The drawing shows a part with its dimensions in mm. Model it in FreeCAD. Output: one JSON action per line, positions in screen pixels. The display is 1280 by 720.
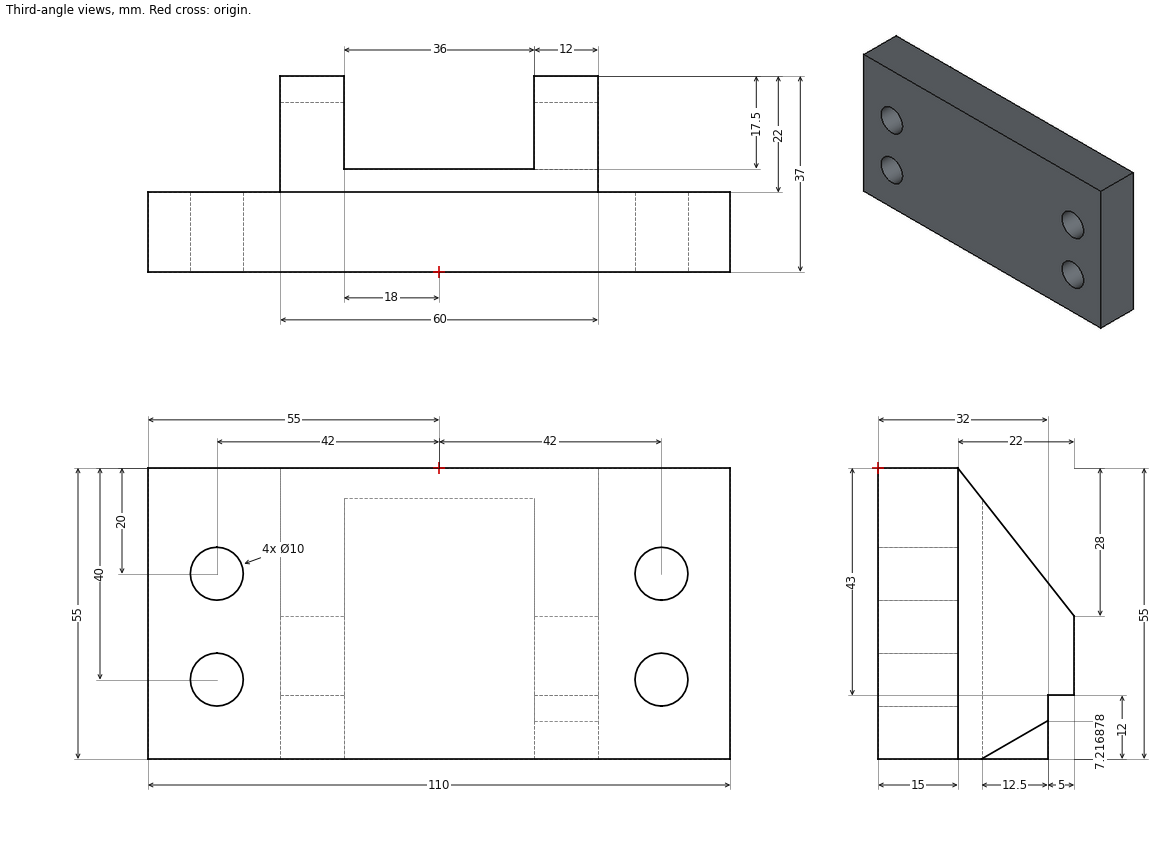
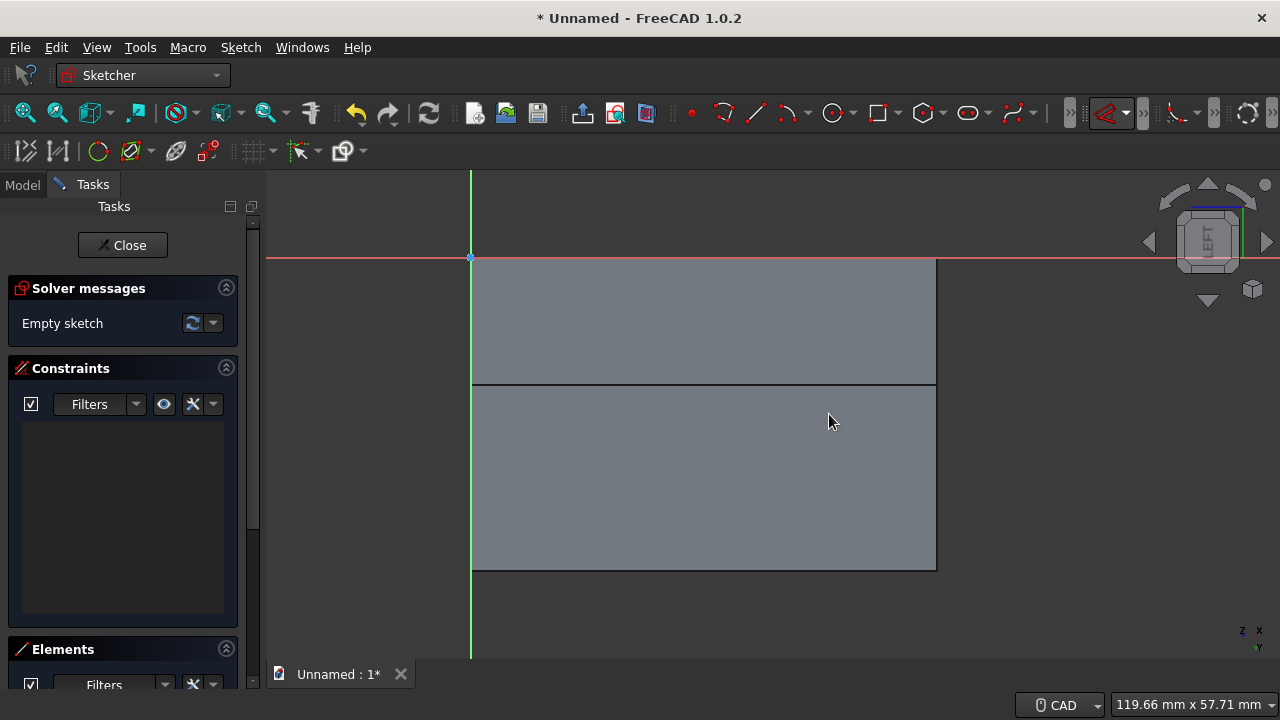
{"action": "left_click", "coordinate": [724, 114]}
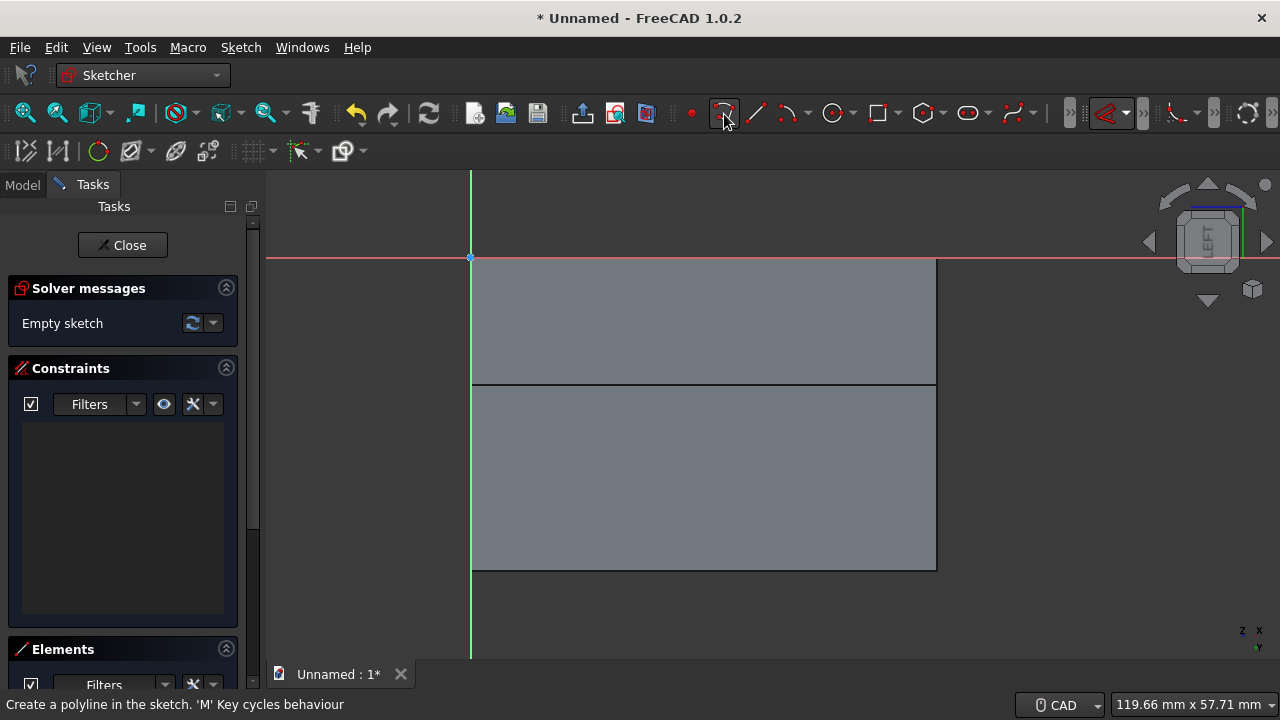
{"action": "left_click", "coordinate": [471, 385]}
{"action": "left_click", "coordinate": [480, 571]}
{"action": "left_click", "coordinate": [708, 571]}
{"action": "left_click", "coordinate": [471, 386]}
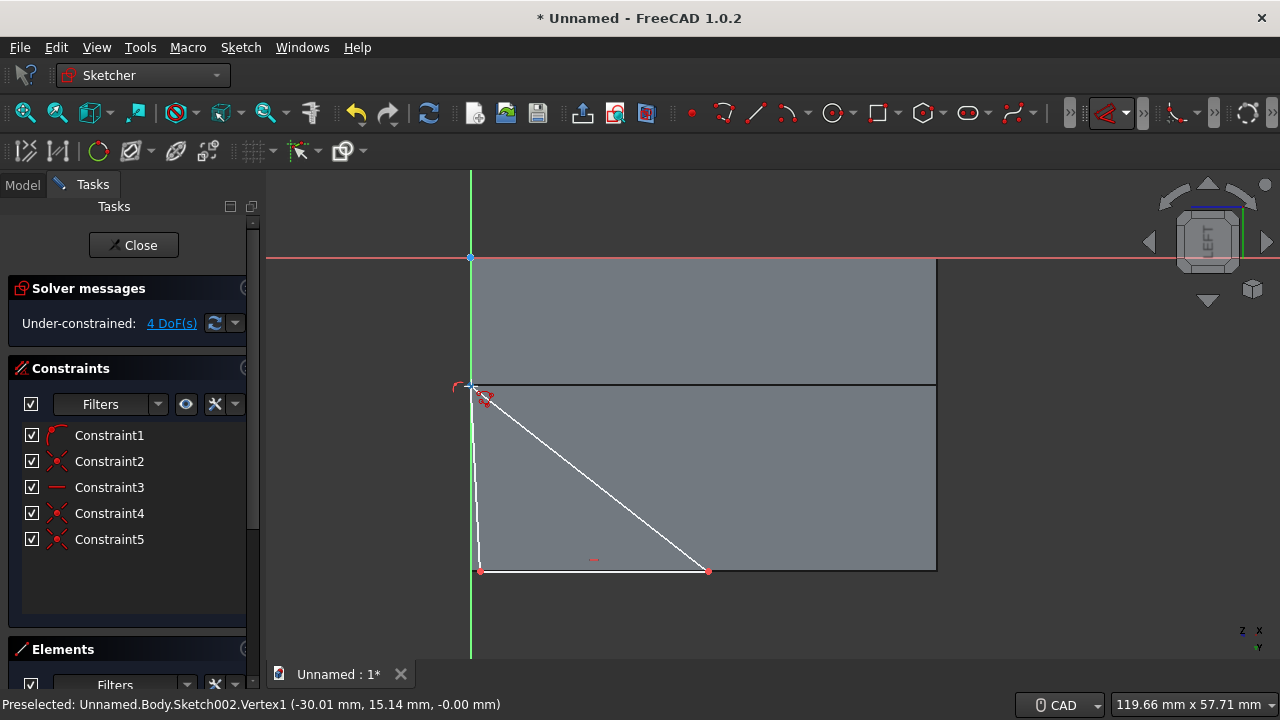
{"action": "left_click", "coordinate": [878, 114]}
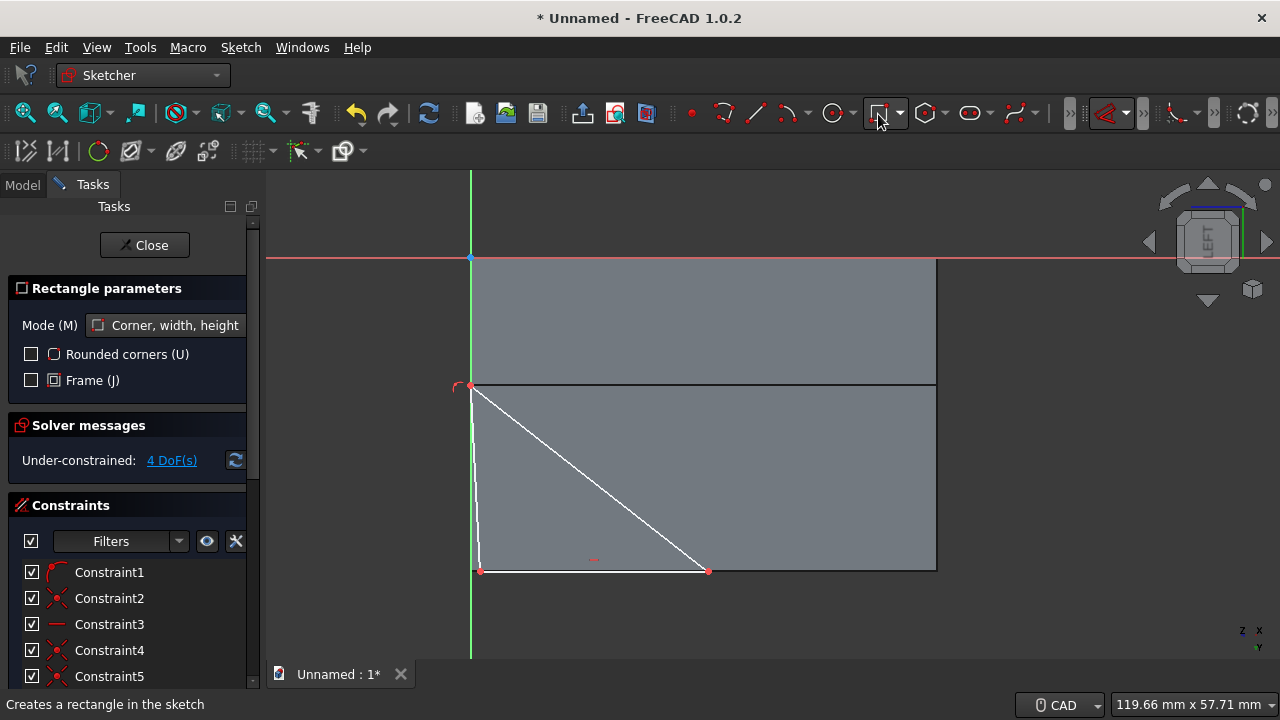
{"action": "left_click", "coordinate": [835, 529]}
{"action": "left_click", "coordinate": [937, 571]}
{"action": "key", "text": "Escape"}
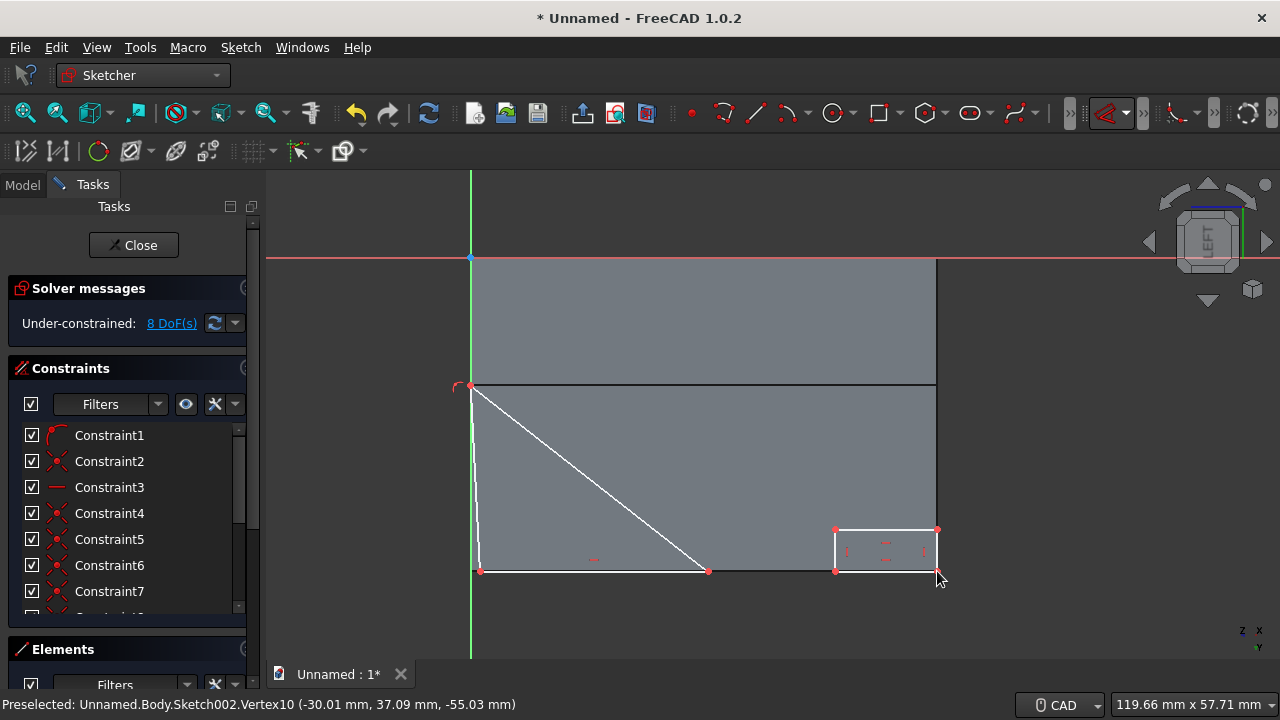
{"action": "left_click", "coordinate": [473, 442]}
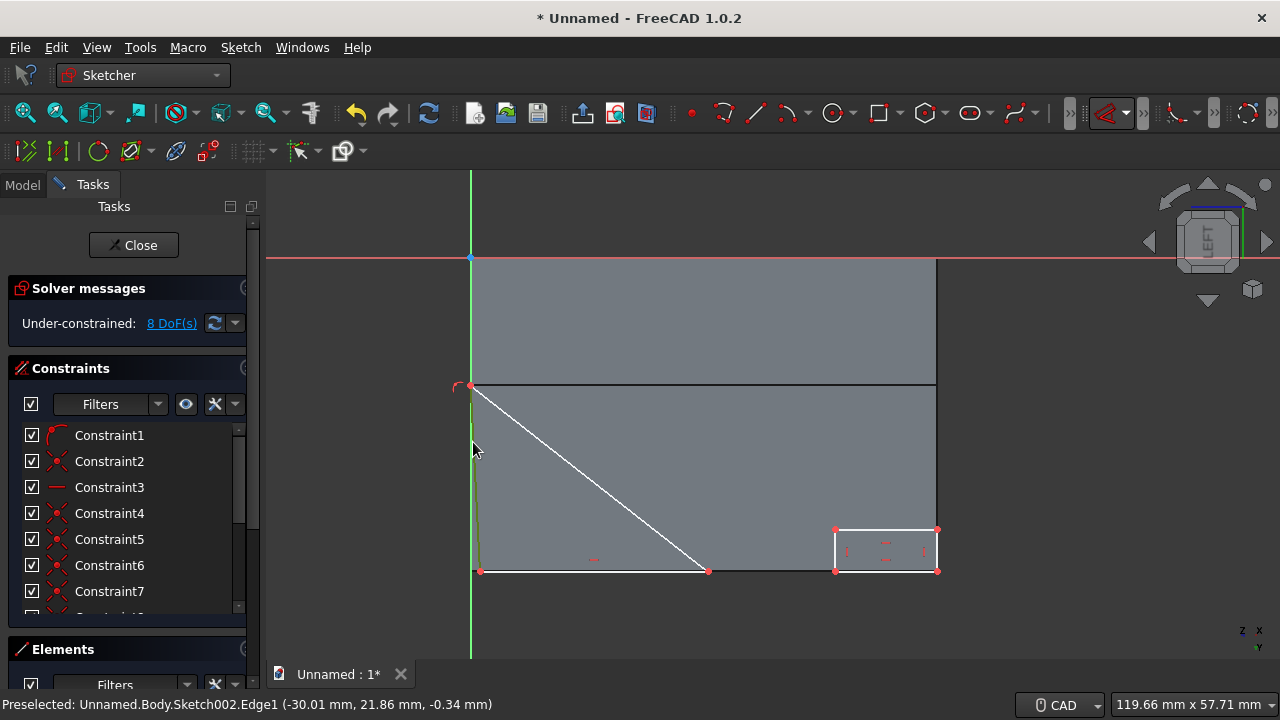
{"action": "key", "text": "v"}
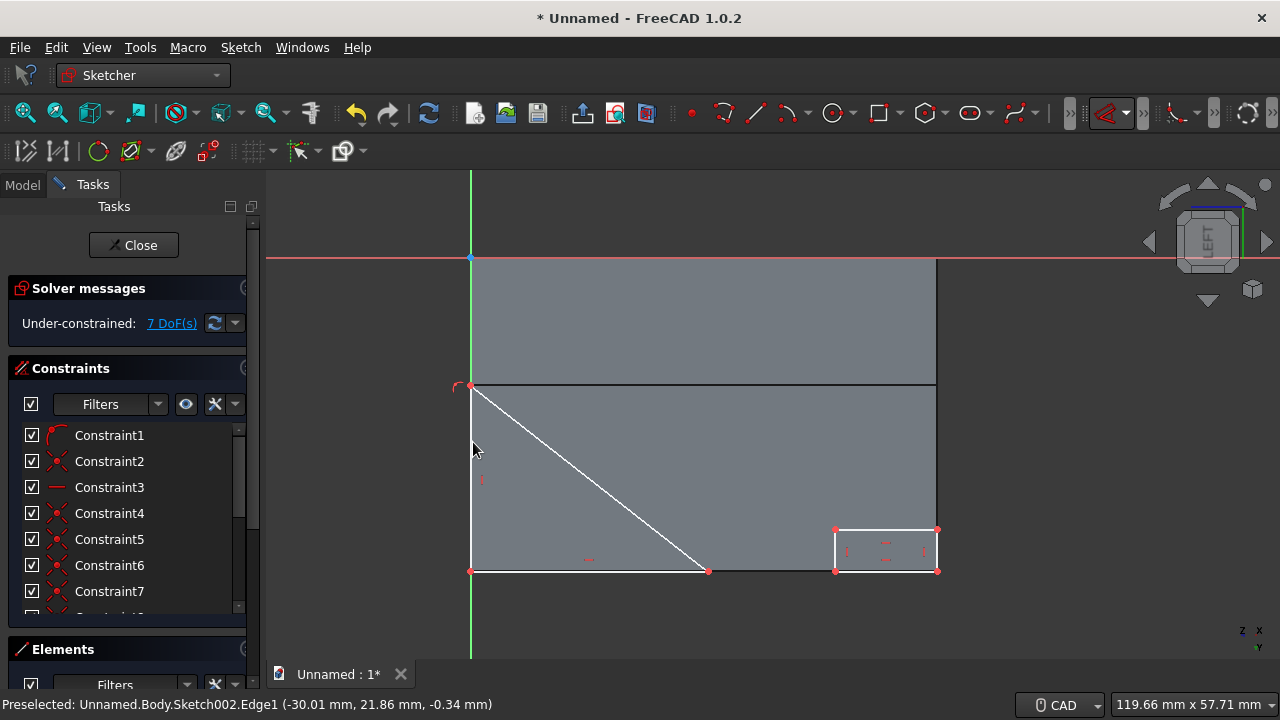
{"action": "left_click", "coordinate": [835, 543]}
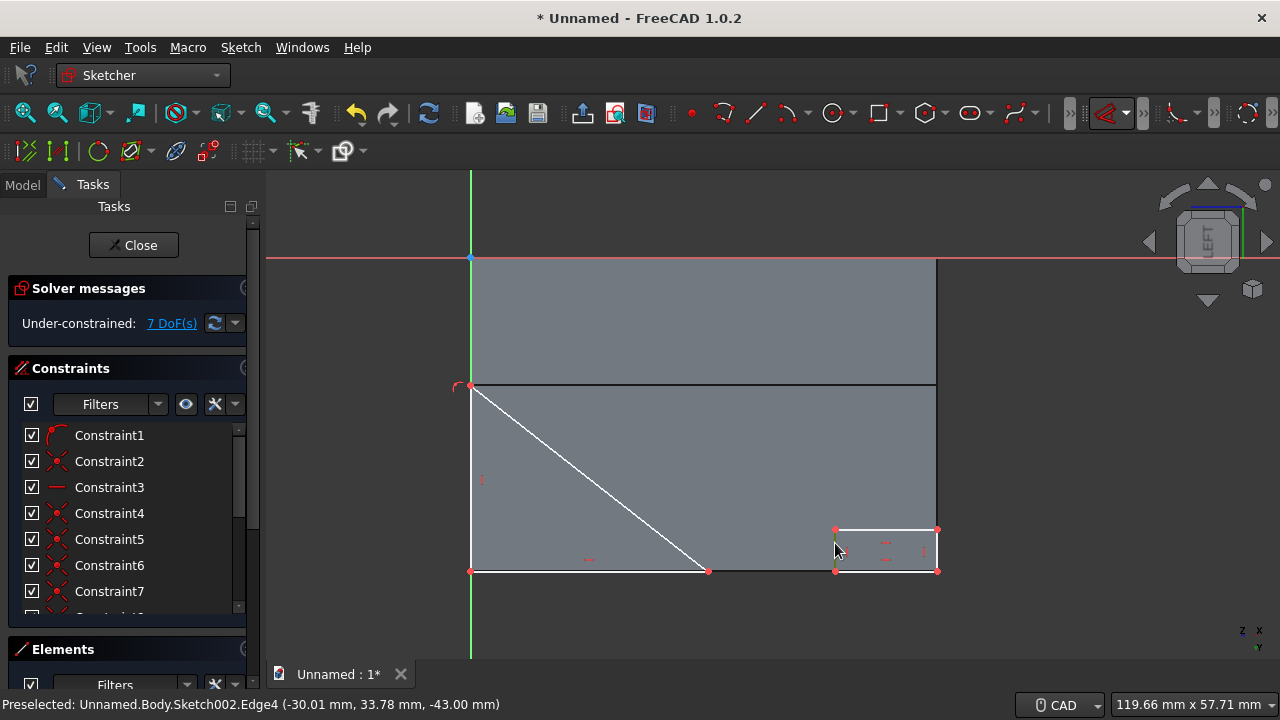
{"action": "left_click", "coordinate": [1128, 114]}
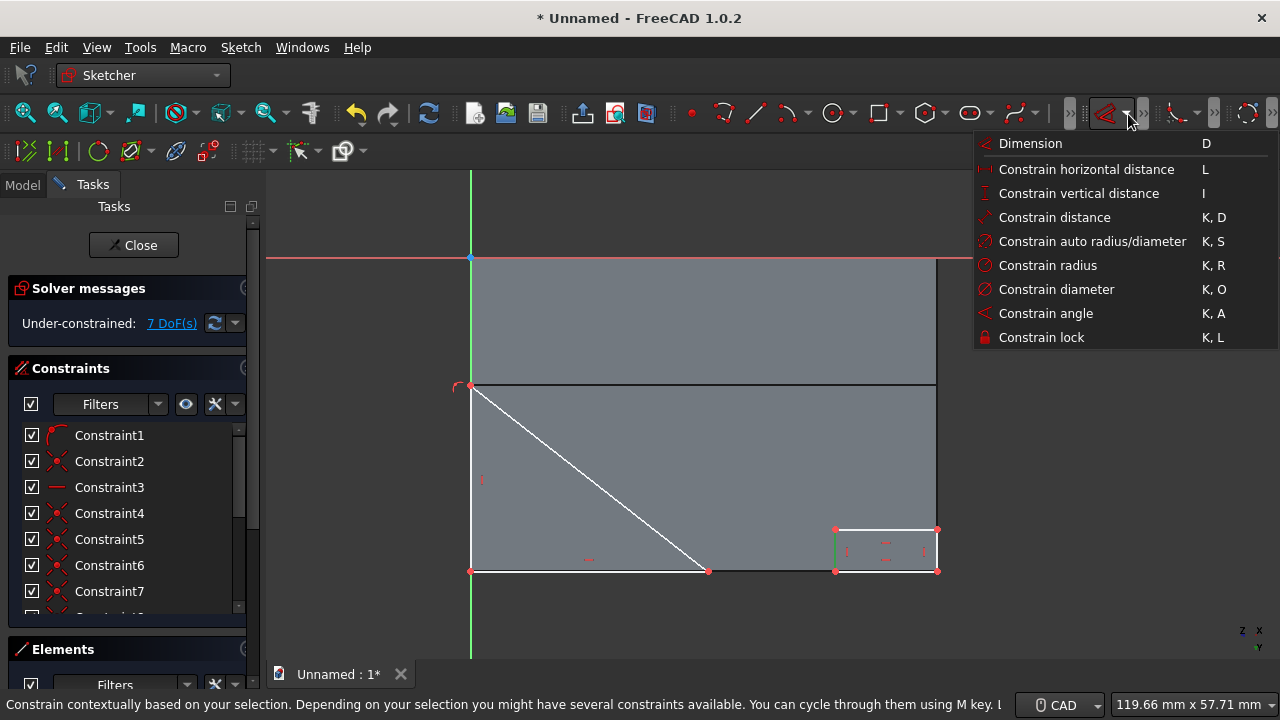
{"action": "left_click", "coordinate": [1126, 193]}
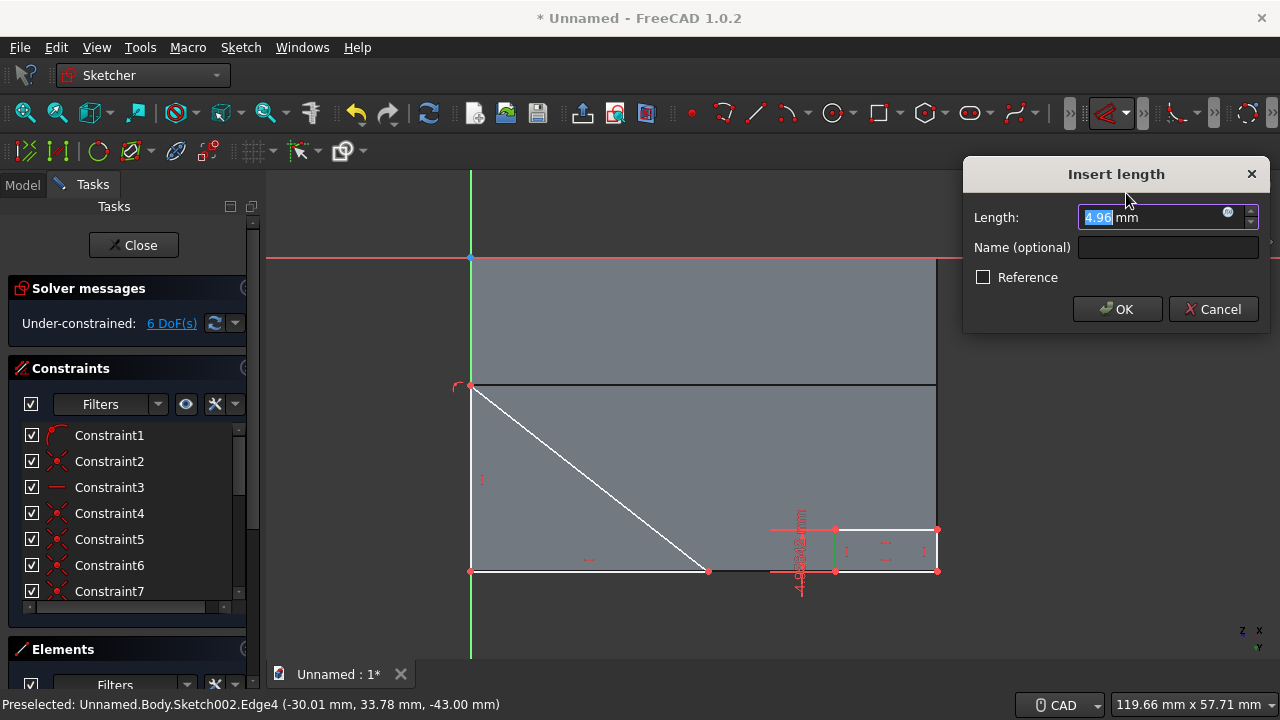
{"action": "type", "text": "5"}
{"action": "key", "text": "Return"}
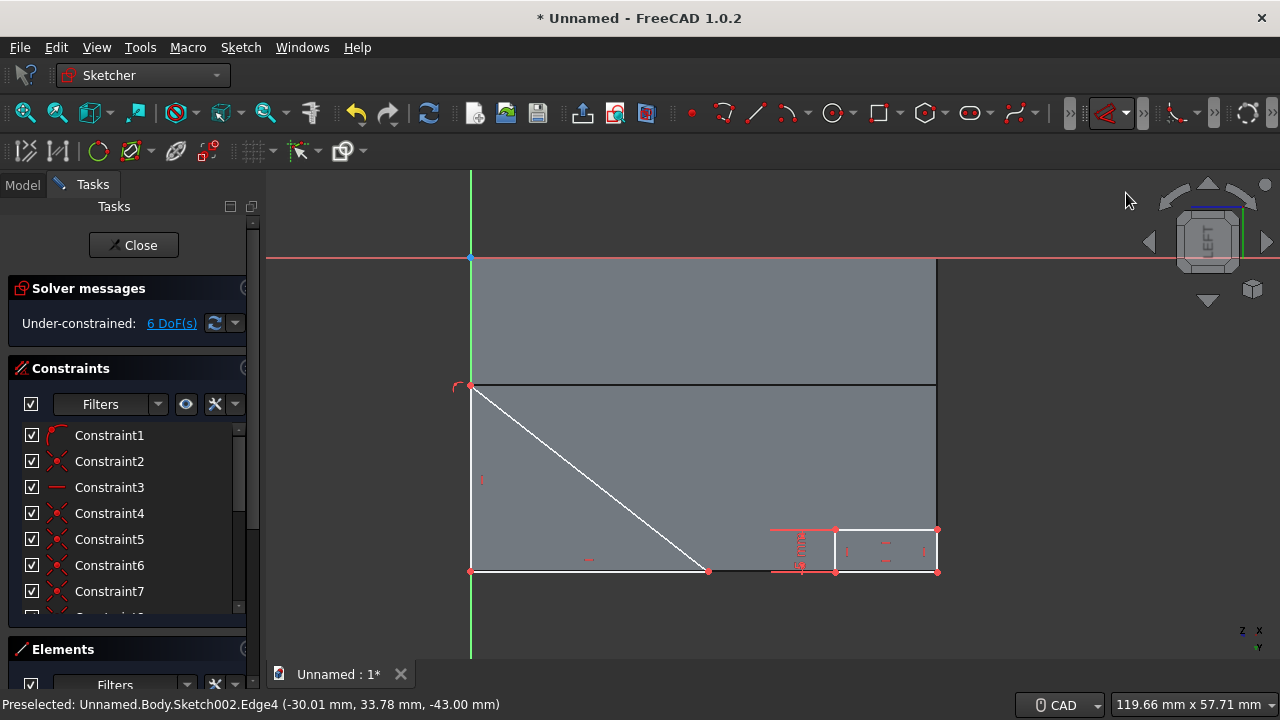
{"action": "left_click", "coordinate": [471, 442]}